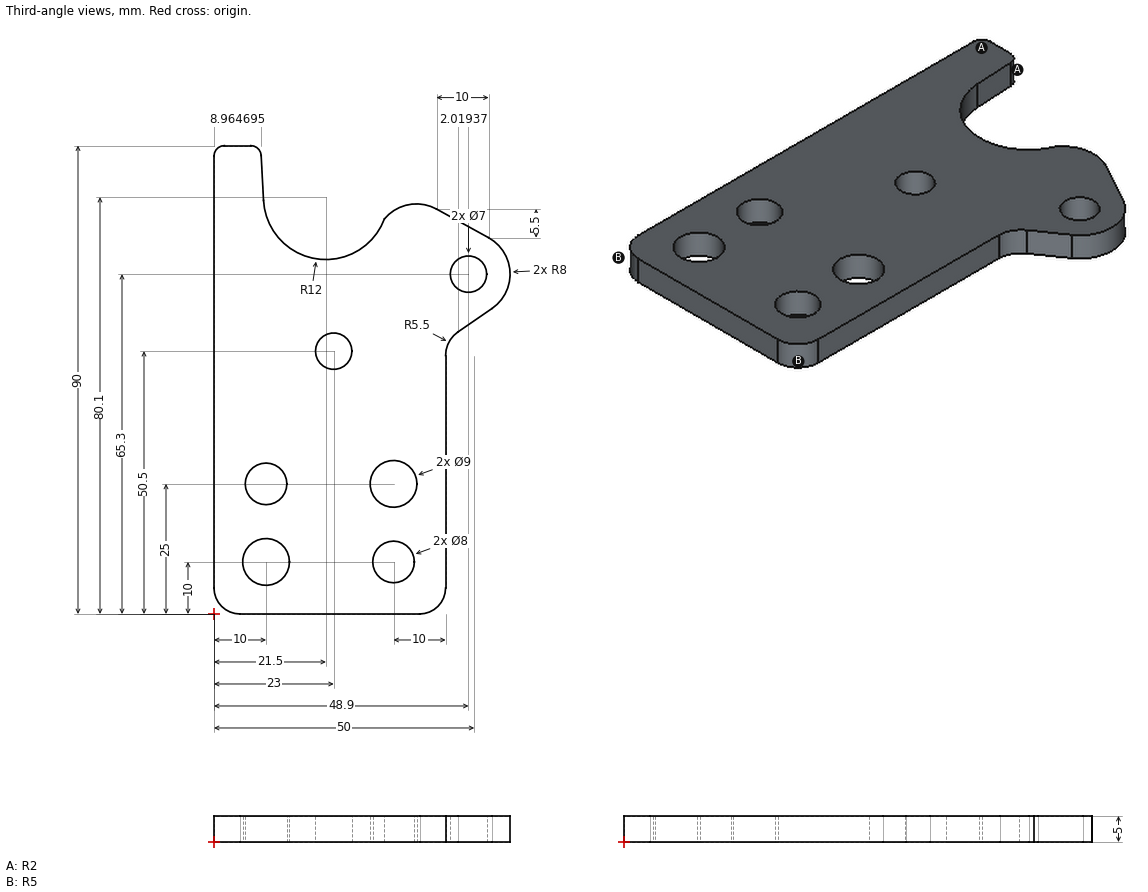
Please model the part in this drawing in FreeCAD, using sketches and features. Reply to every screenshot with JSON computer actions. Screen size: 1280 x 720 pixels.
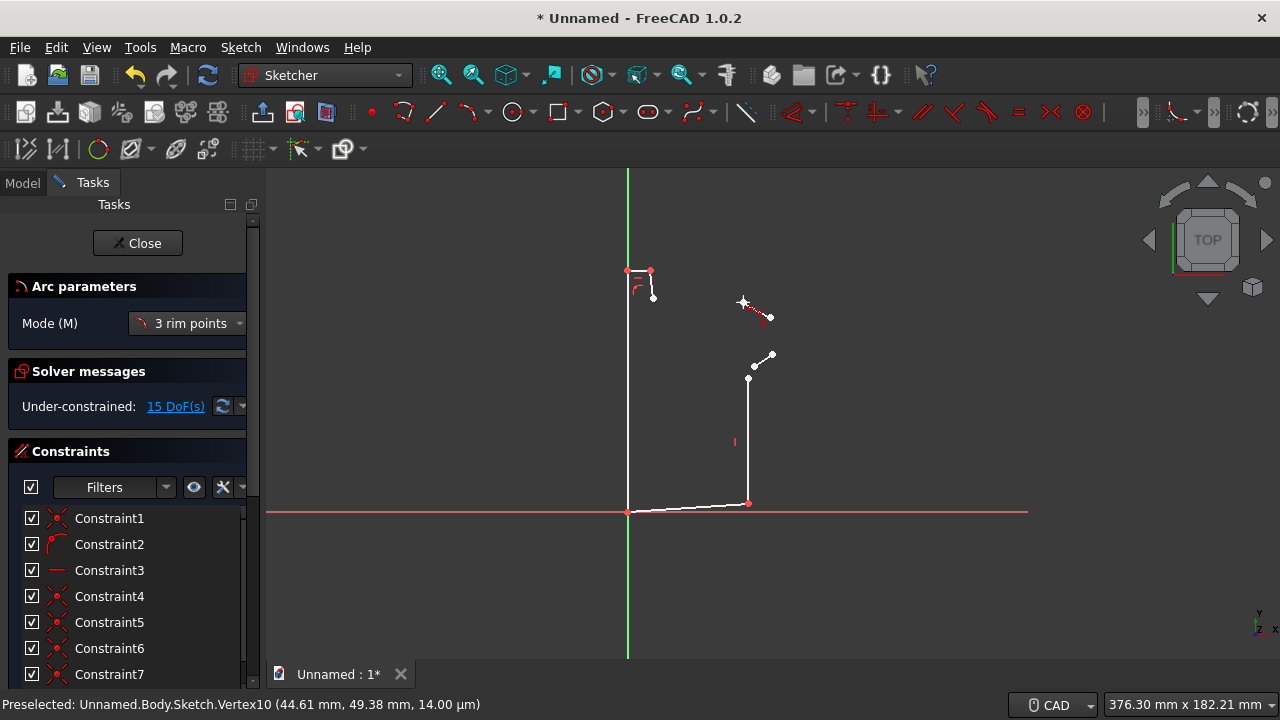
{"action": "left_click", "coordinate": [748, 379]}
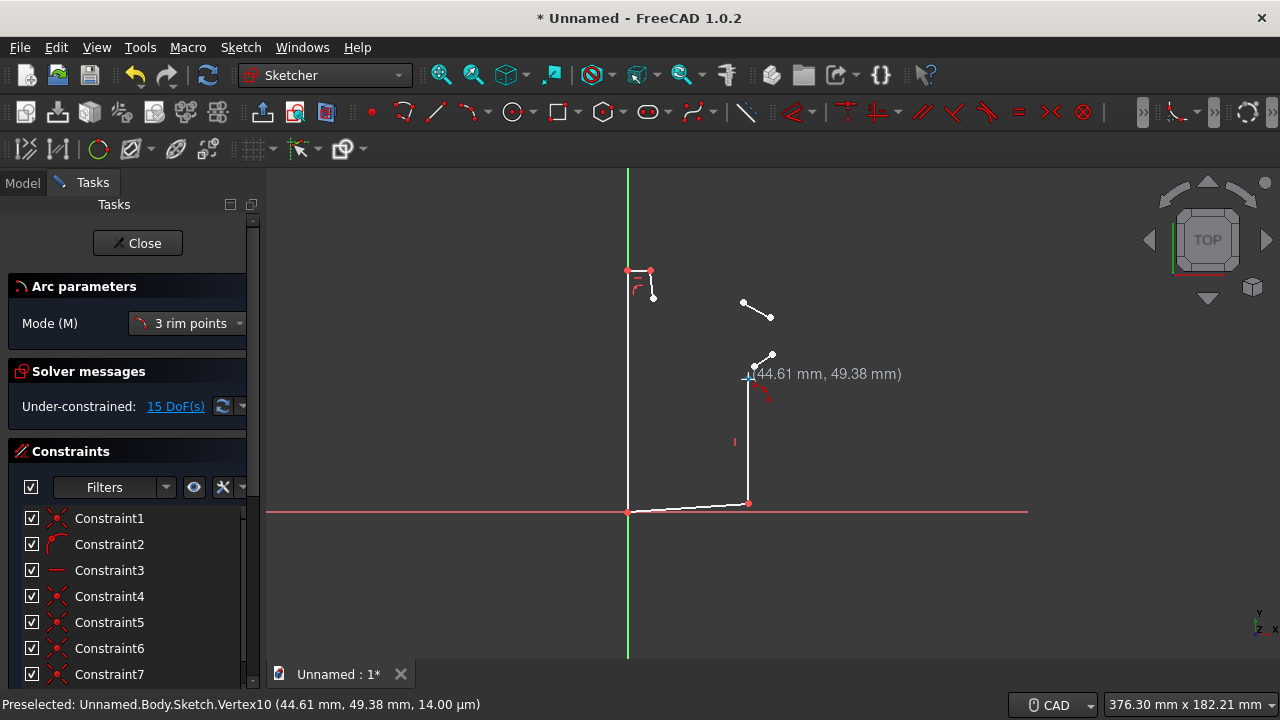
{"action": "scroll", "coordinate": [754, 366], "scroll_direction": "up", "scroll_amount": 2}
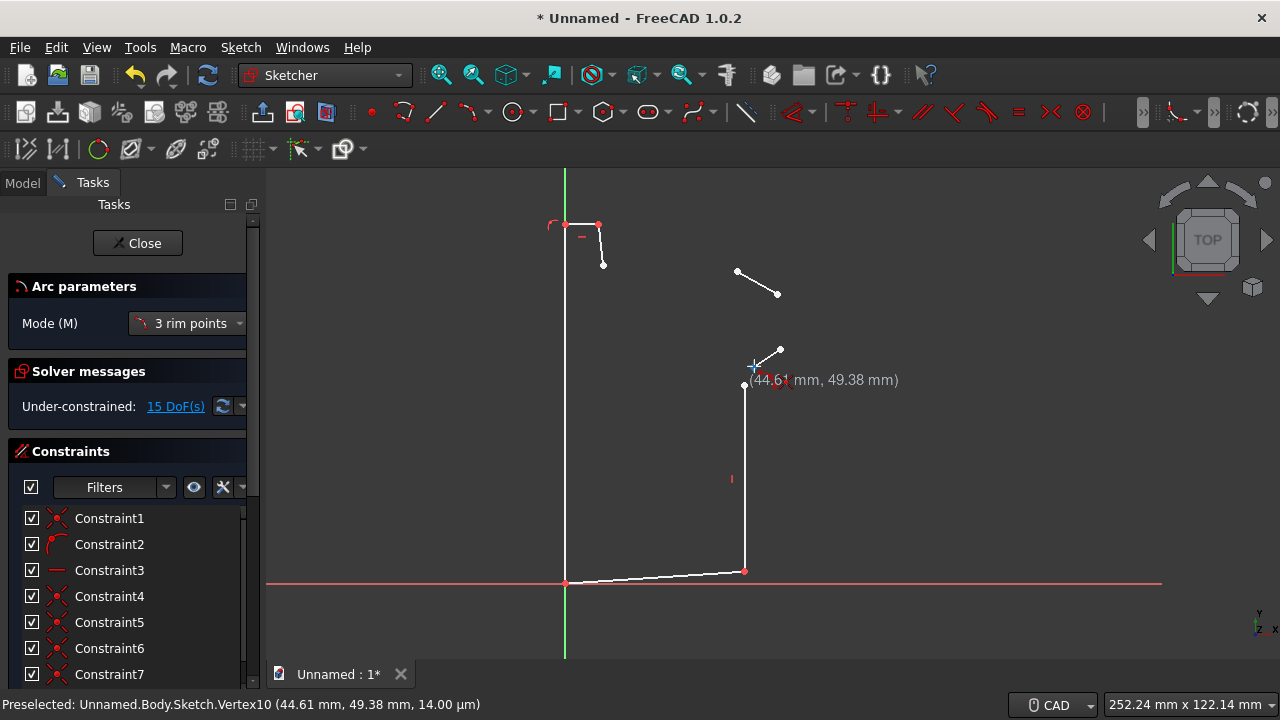
{"action": "left_click", "coordinate": [754, 367]}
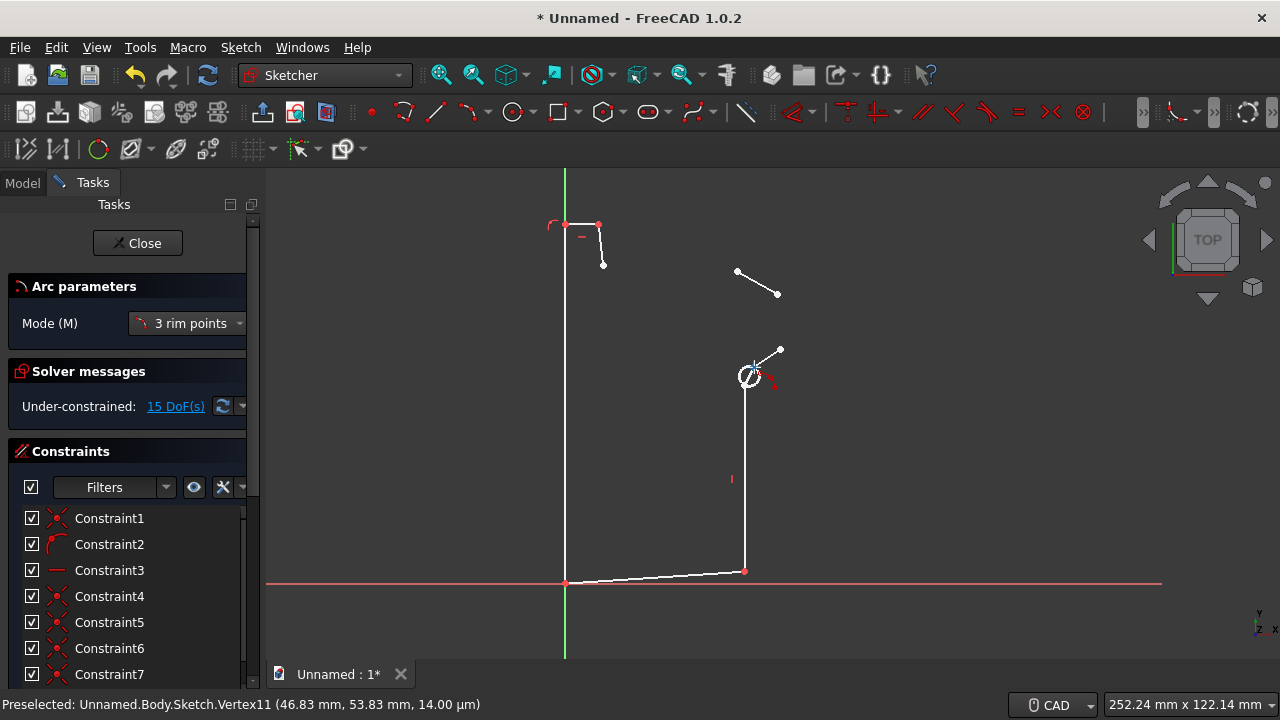
{"action": "scroll", "coordinate": [747, 374], "scroll_direction": "up", "scroll_amount": 10}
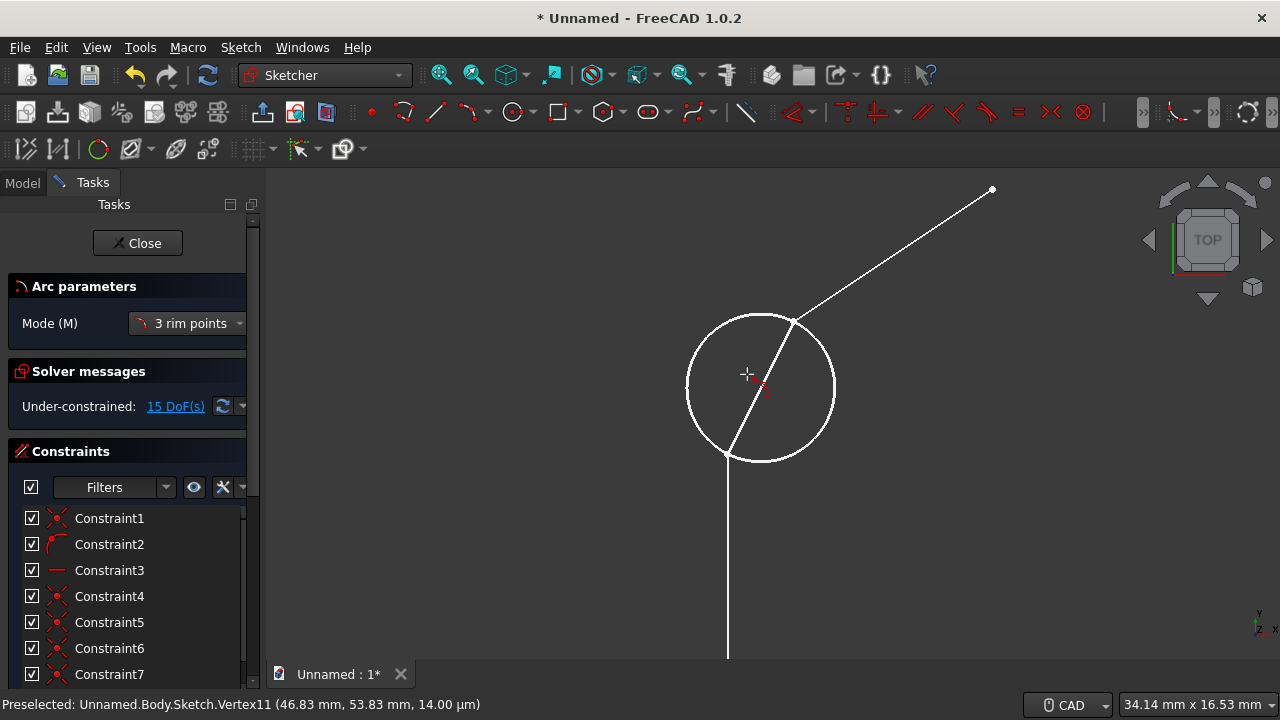
{"action": "left_click", "coordinate": [743, 370]}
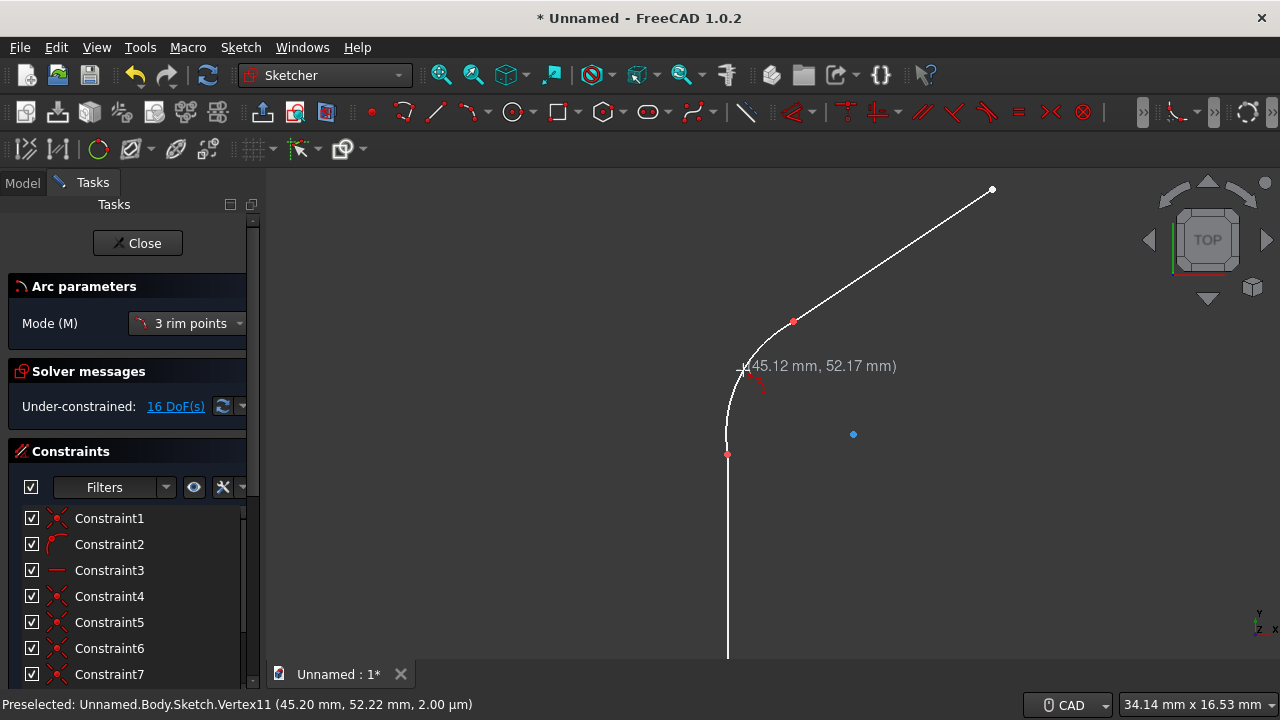
{"action": "scroll", "coordinate": [761, 392], "scroll_direction": "down", "scroll_amount": 11}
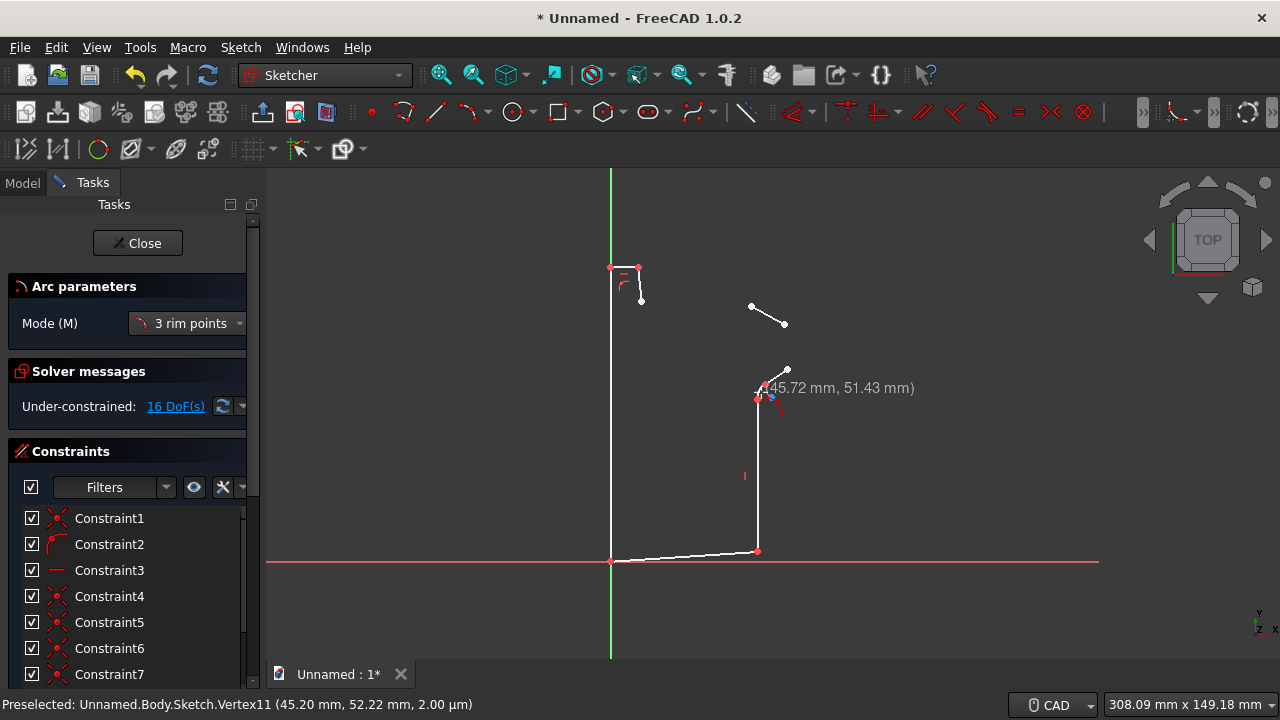
{"action": "left_click", "coordinate": [787, 370]}
{"action": "left_click", "coordinate": [785, 325]}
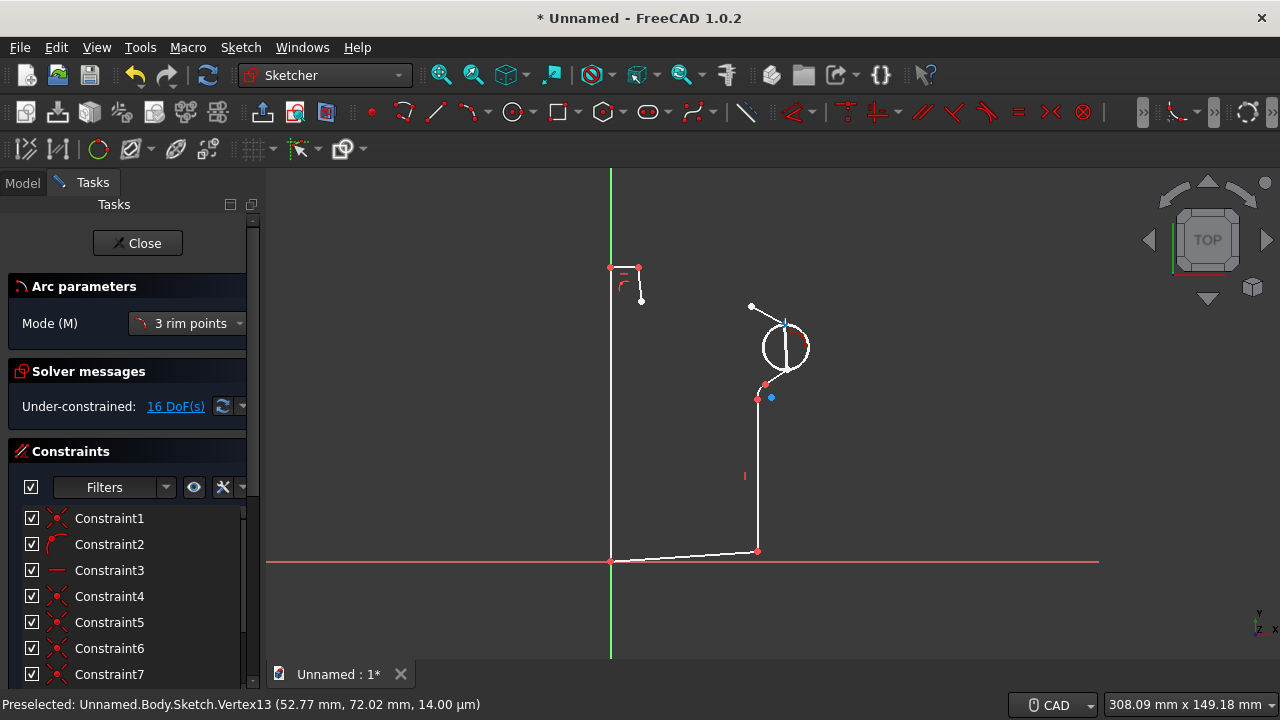
{"action": "scroll", "coordinate": [798, 346], "scroll_direction": "up", "scroll_amount": 2}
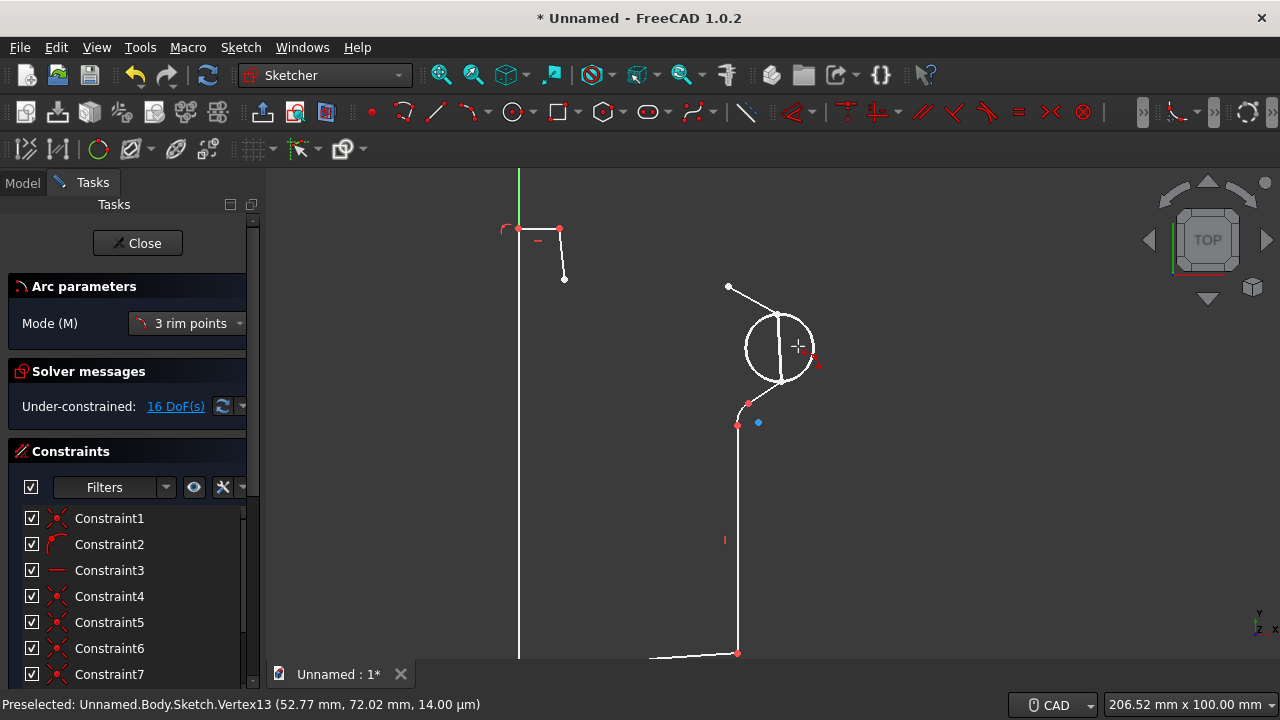
{"action": "left_click", "coordinate": [798, 345]}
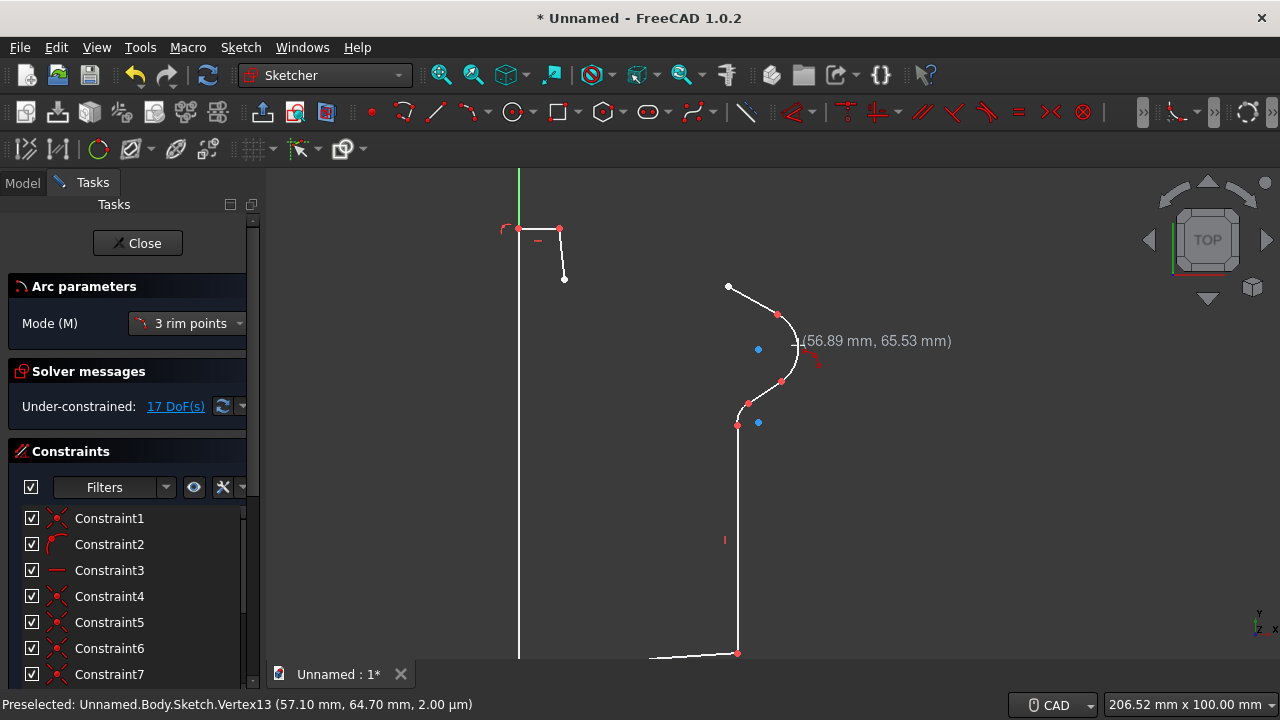
{"action": "left_click", "coordinate": [729, 287]}
{"action": "left_click", "coordinate": [679, 295]}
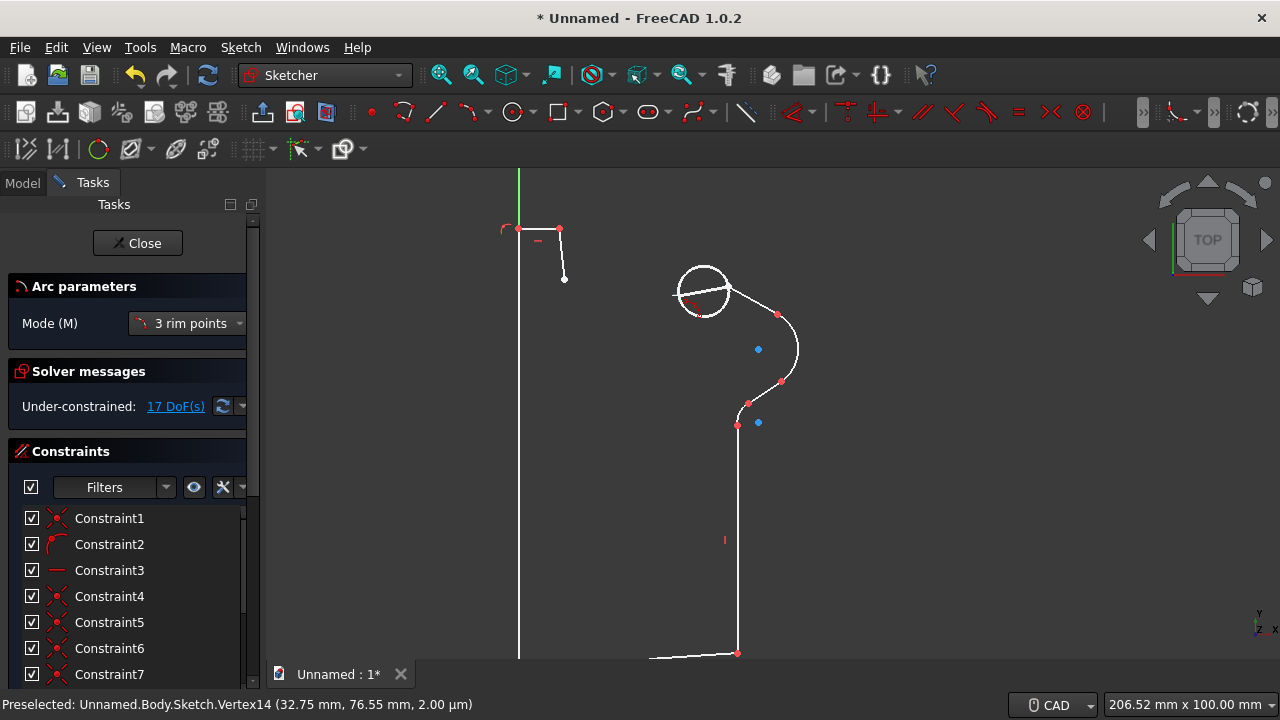
{"action": "scroll", "coordinate": [702, 282], "scroll_direction": "up", "scroll_amount": 3}